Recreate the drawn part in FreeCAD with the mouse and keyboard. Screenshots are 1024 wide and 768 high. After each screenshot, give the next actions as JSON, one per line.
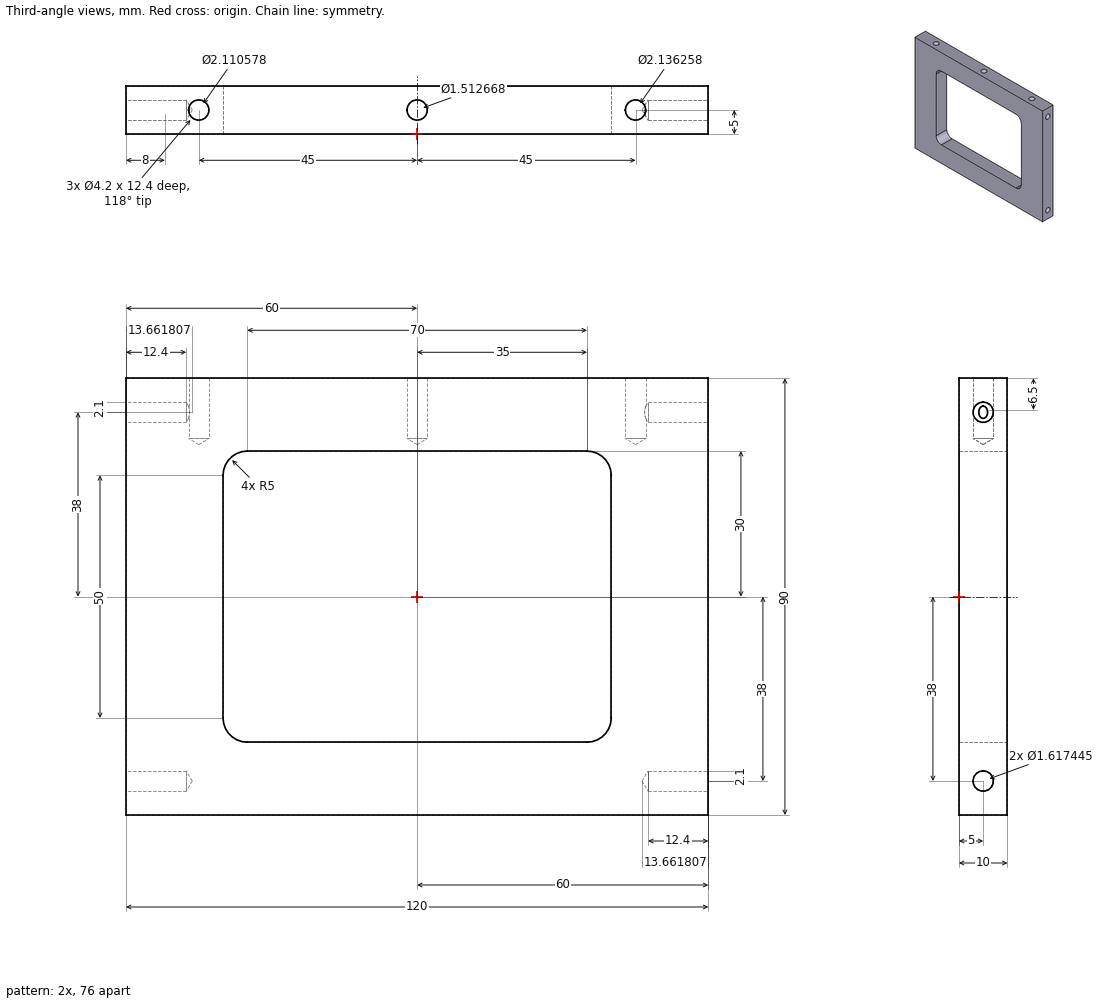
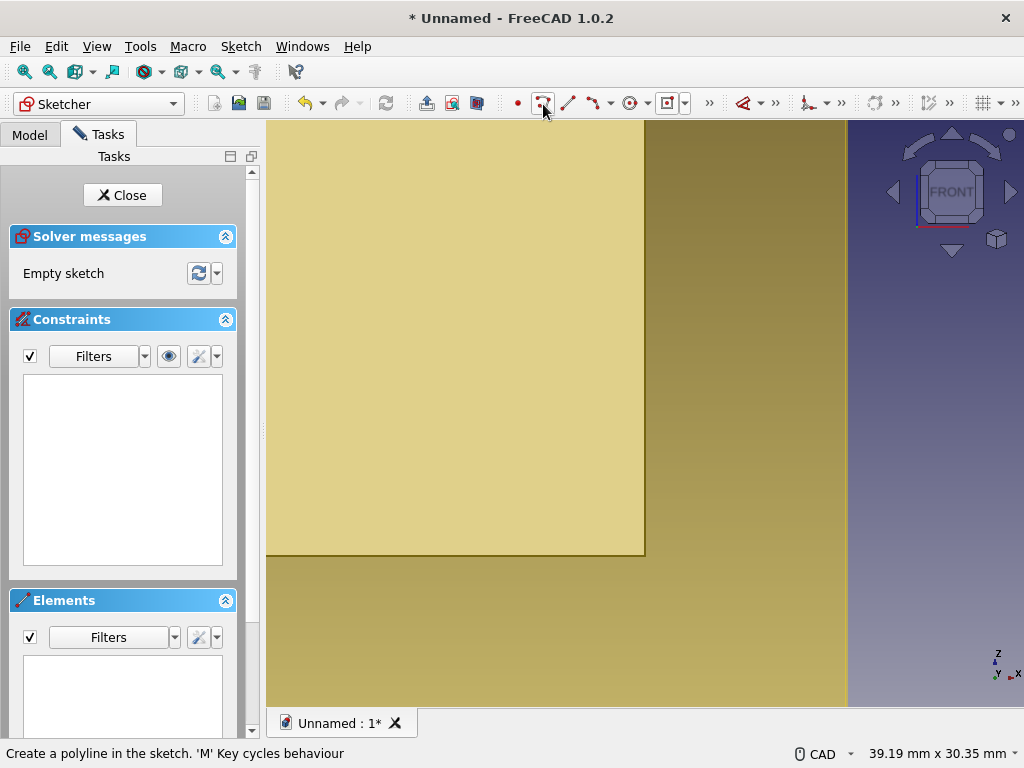
{"action": "left_click", "coordinate": [405, 380]}
{"action": "left_click", "coordinate": [645, 380]}
{"action": "left_click", "coordinate": [645, 420]}
{"action": "left_click", "coordinate": [381, 420]}
{"action": "left_click", "coordinate": [405, 381]}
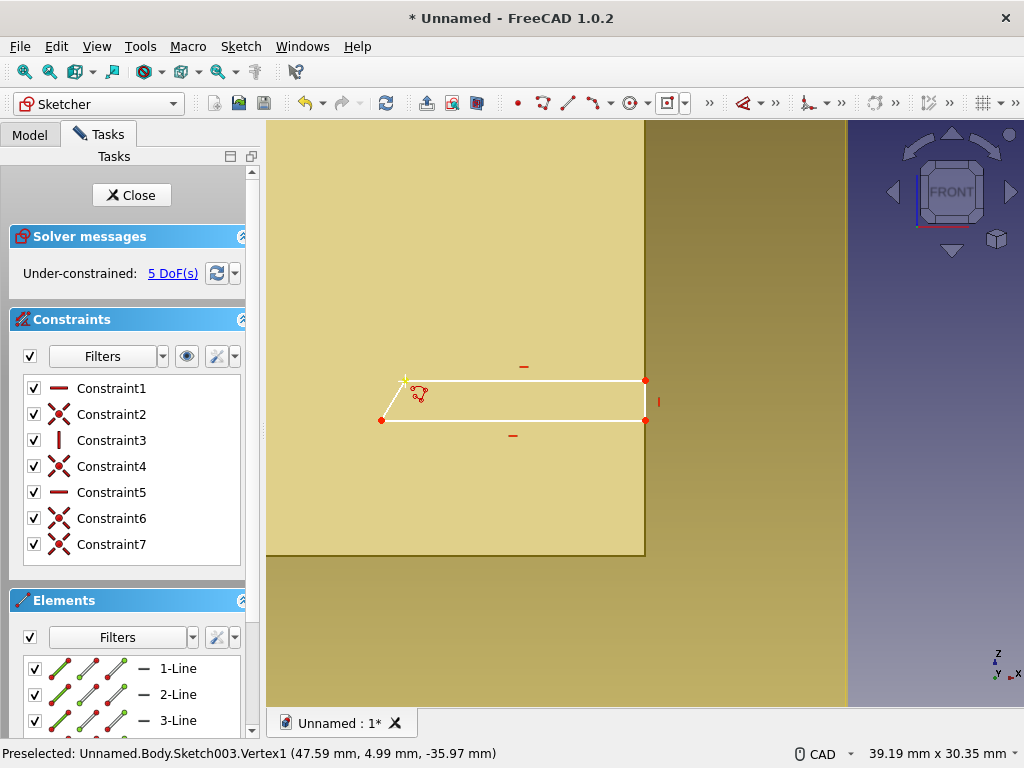
{"action": "left_click", "coordinate": [568, 104]}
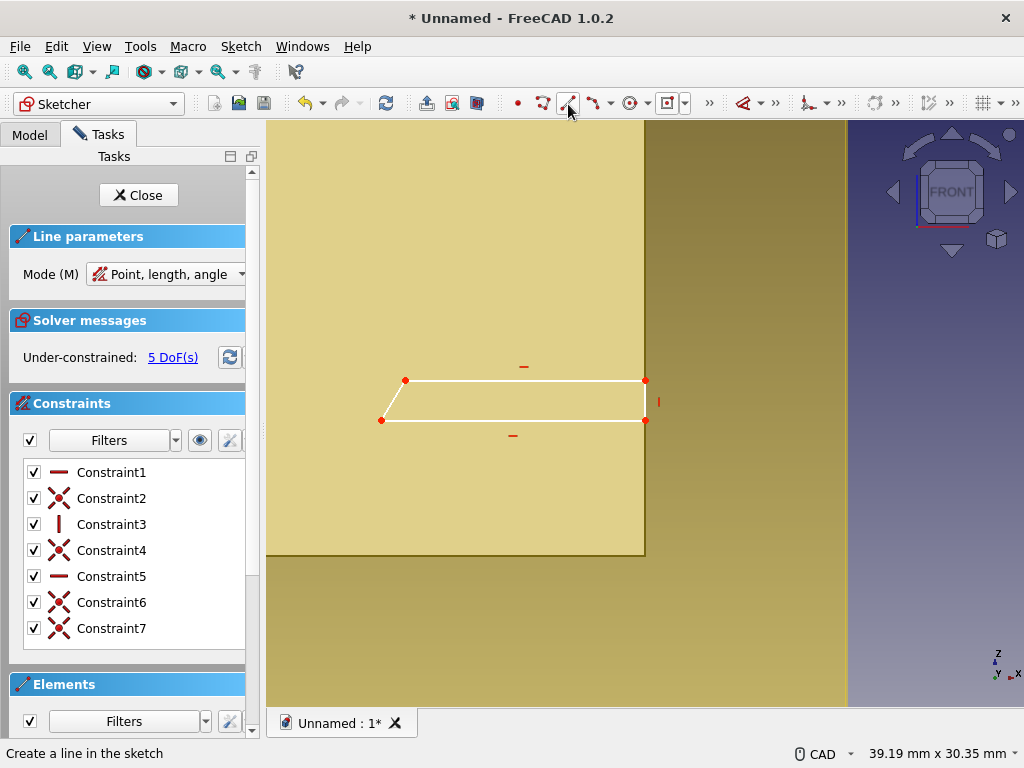
{"action": "left_click", "coordinate": [671, 420]}
{"action": "left_click", "coordinate": [751, 420]}
{"action": "key", "text": "Escape"}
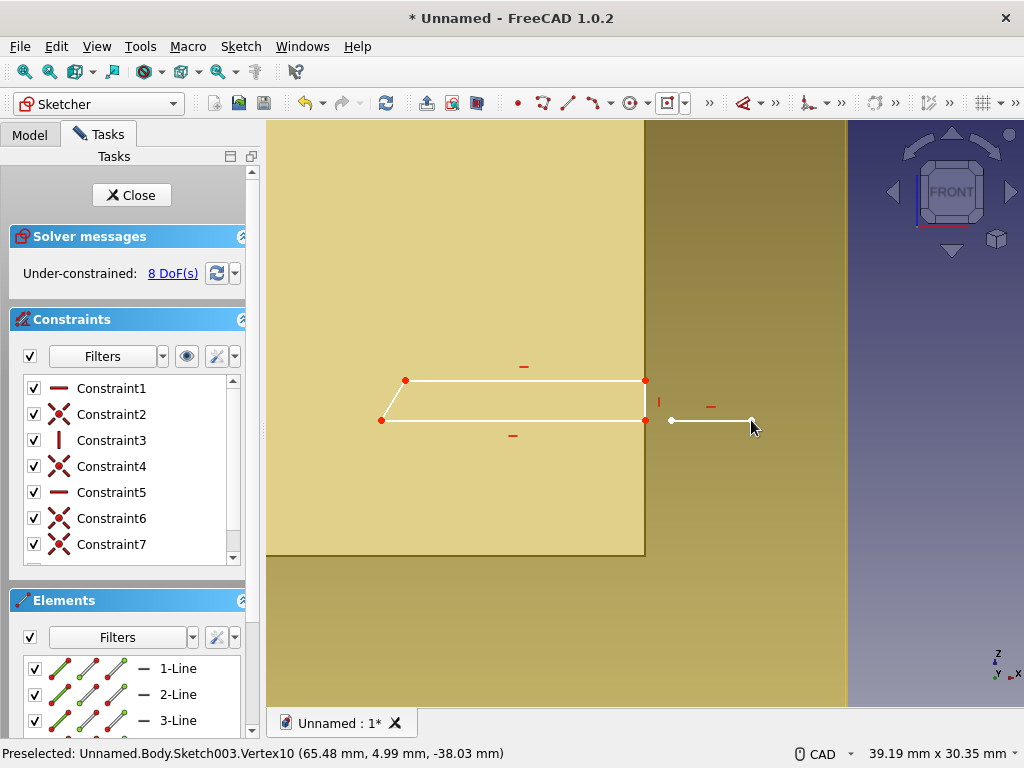
{"action": "left_click", "coordinate": [695, 421]}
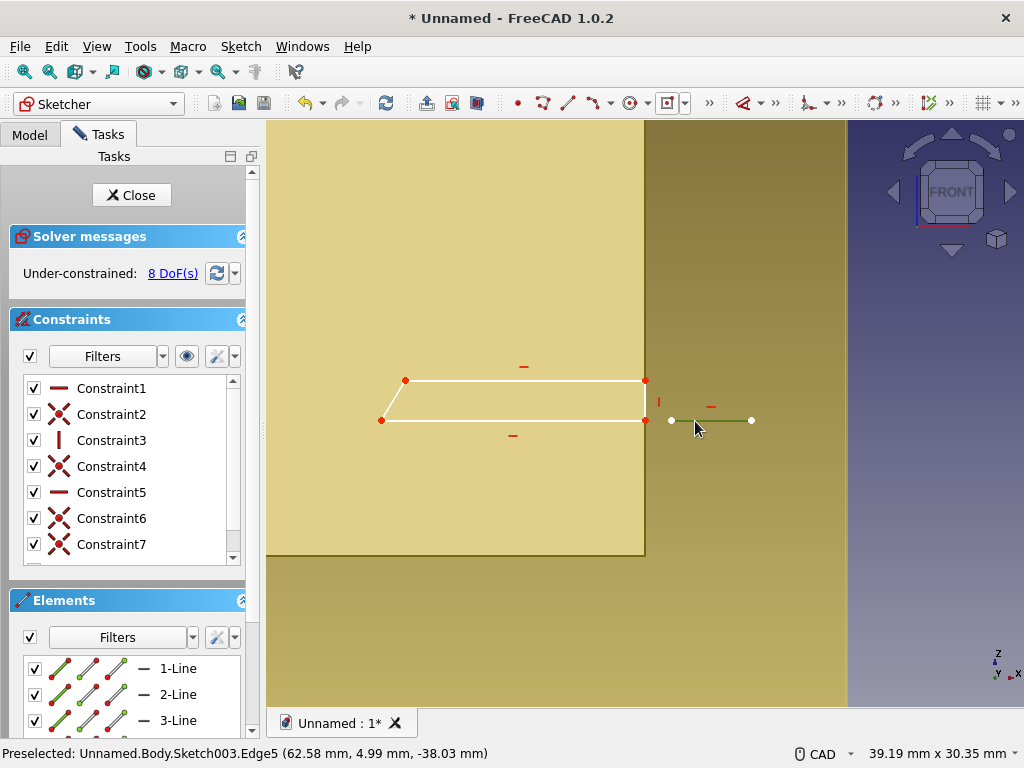
{"action": "key", "text": "g n"}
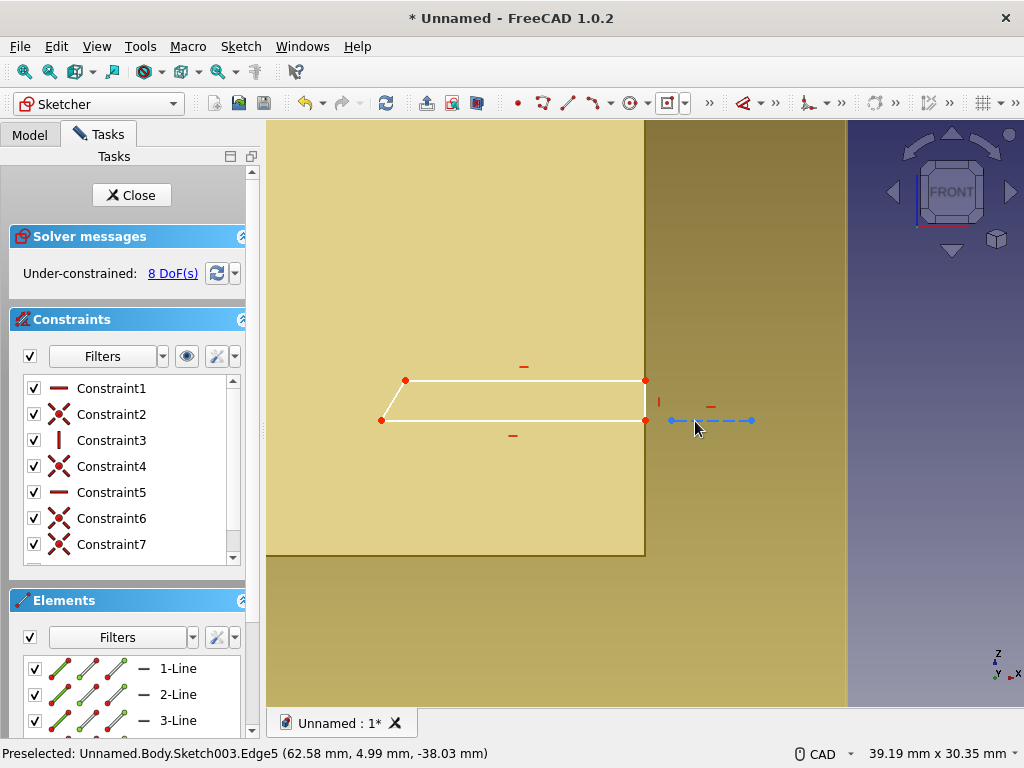
{"action": "left_click", "coordinate": [742, 104]}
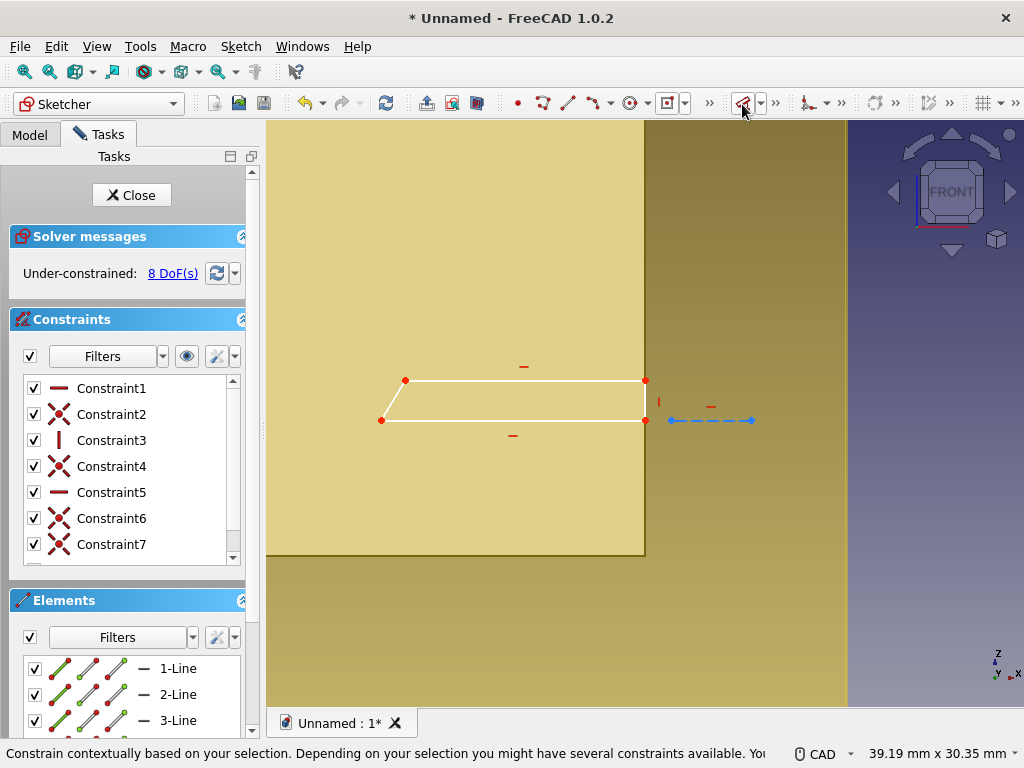
{"action": "left_click", "coordinate": [645, 393]}
{"action": "left_click", "coordinate": [679, 401]}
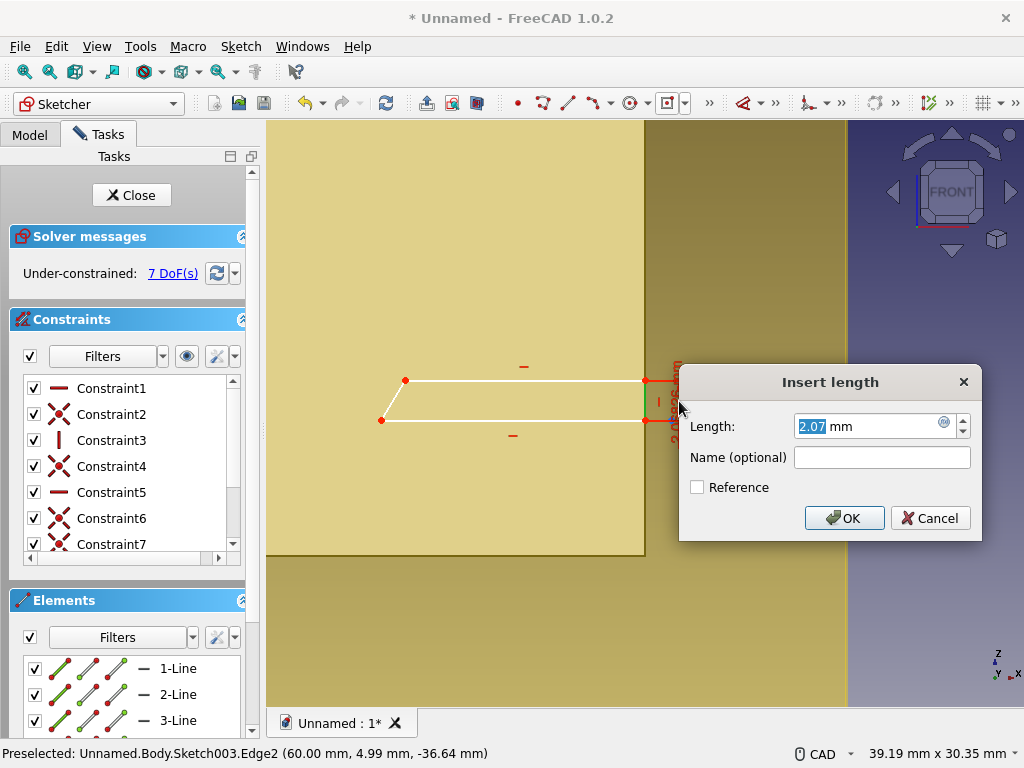
{"action": "type", "text": "2.1"}
{"action": "key", "text": "Return"}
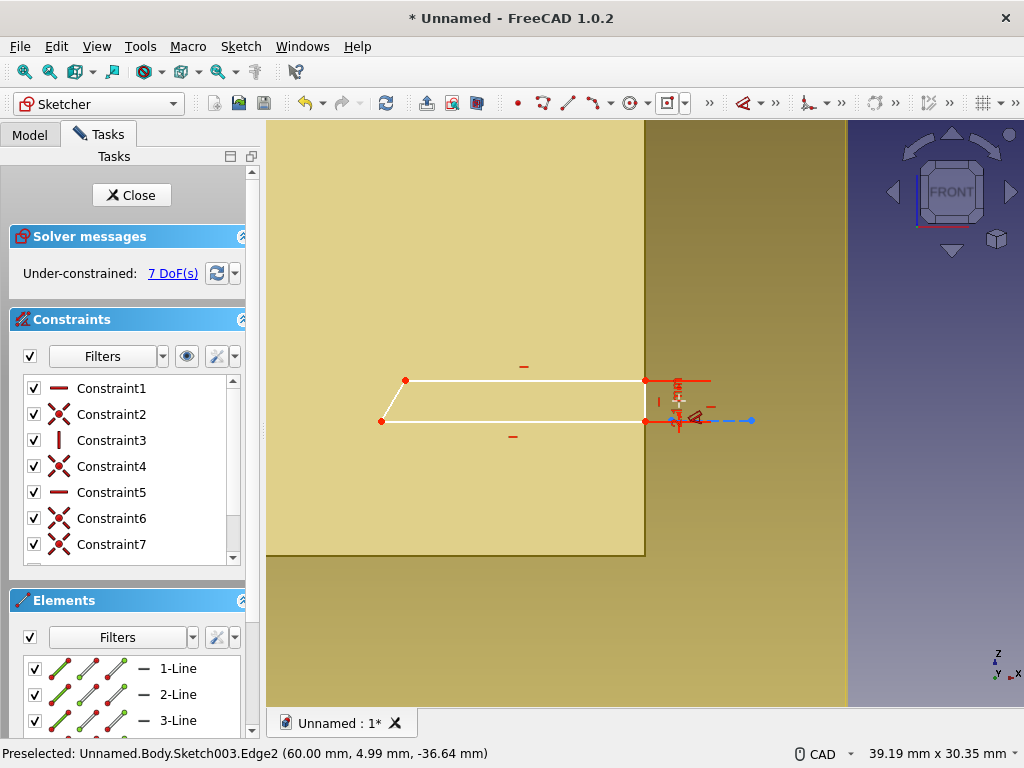
{"action": "left_click", "coordinate": [645, 381]}
{"action": "left_click", "coordinate": [347, 415]}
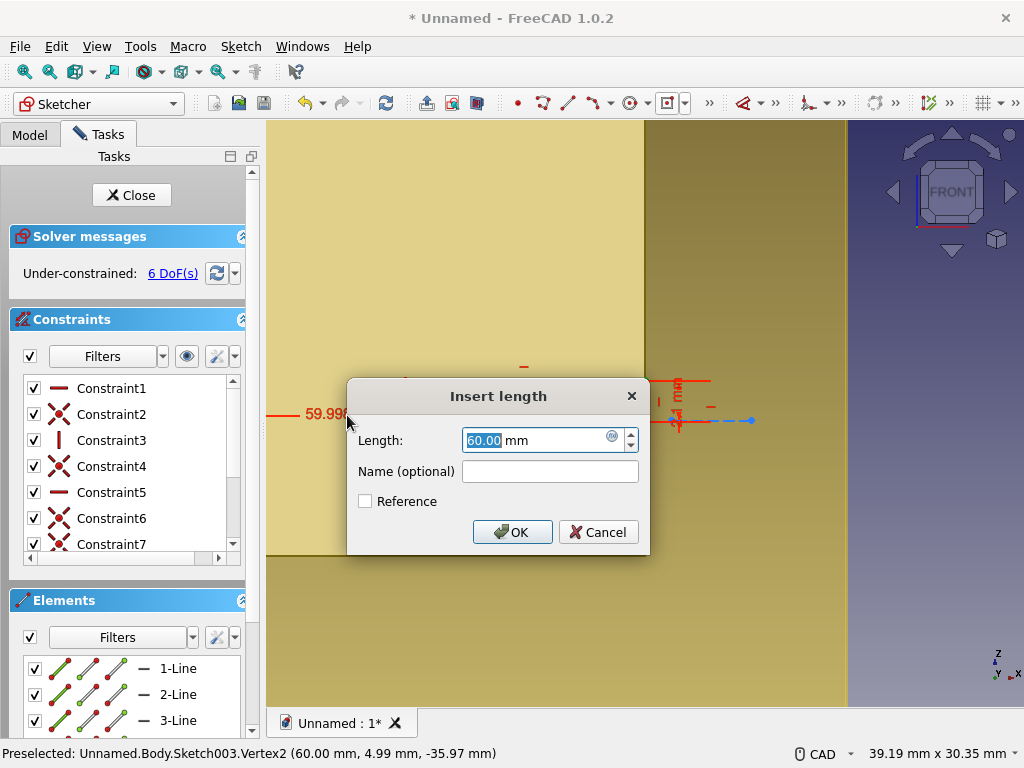
{"action": "type", "text": "60"}
{"action": "key", "text": "Return"}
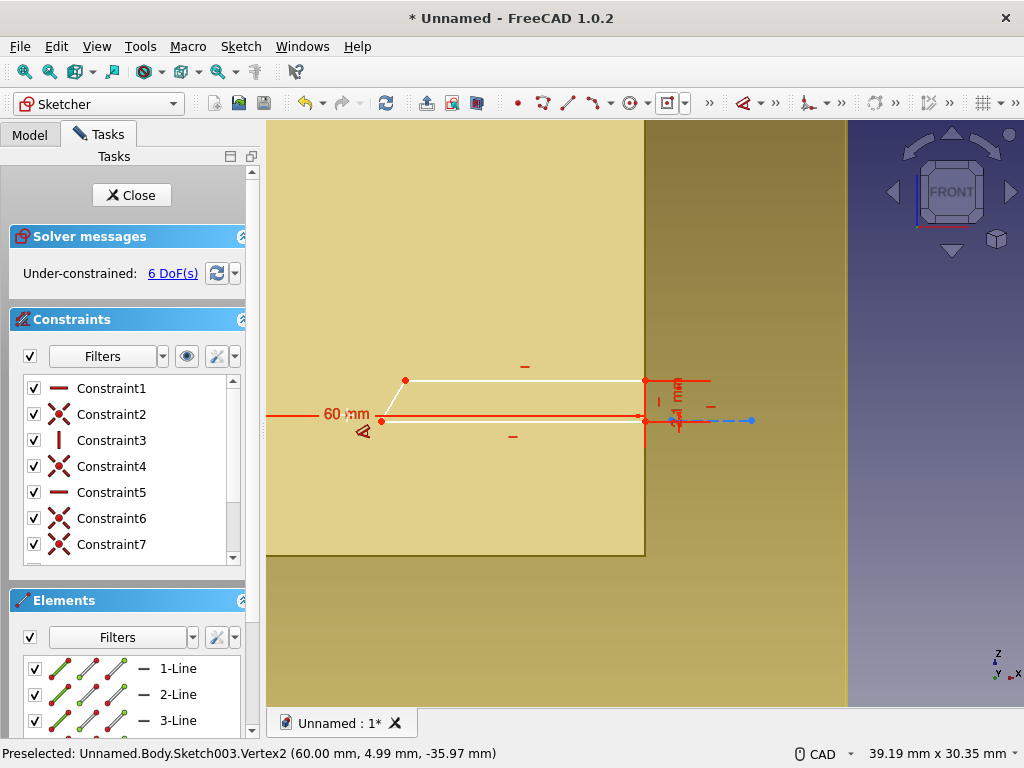
{"action": "left_click", "coordinate": [645, 422]}
{"action": "left_click", "coordinate": [679, 285]}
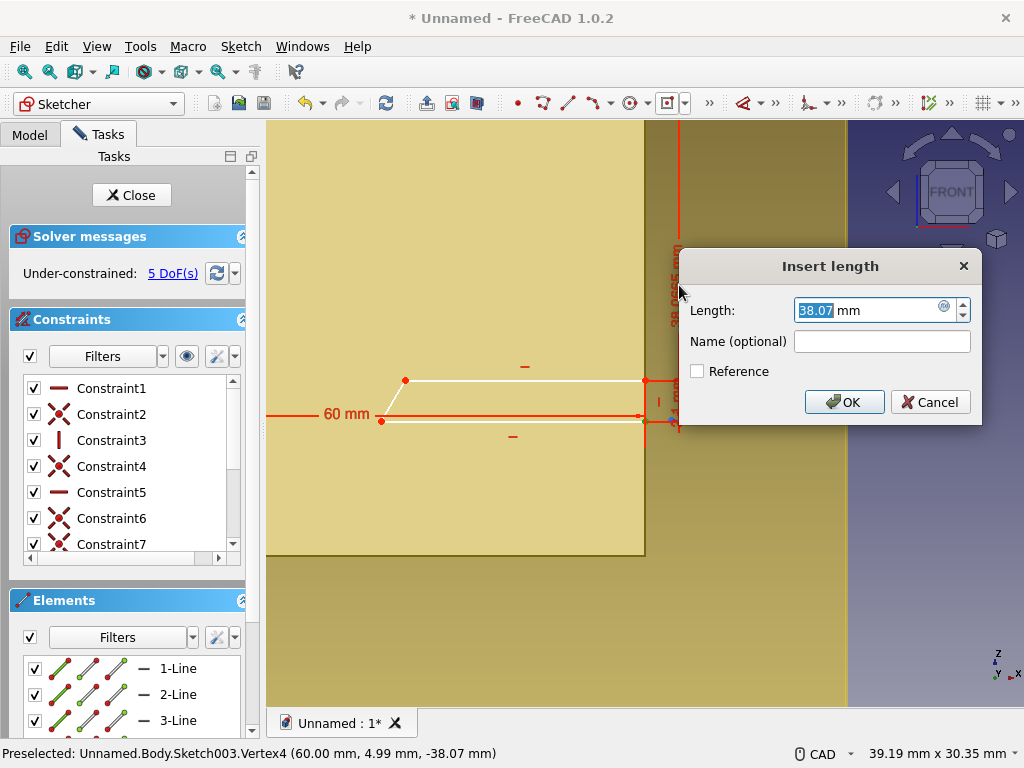
{"action": "type", "text": "38"}
{"action": "key", "text": "Return"}